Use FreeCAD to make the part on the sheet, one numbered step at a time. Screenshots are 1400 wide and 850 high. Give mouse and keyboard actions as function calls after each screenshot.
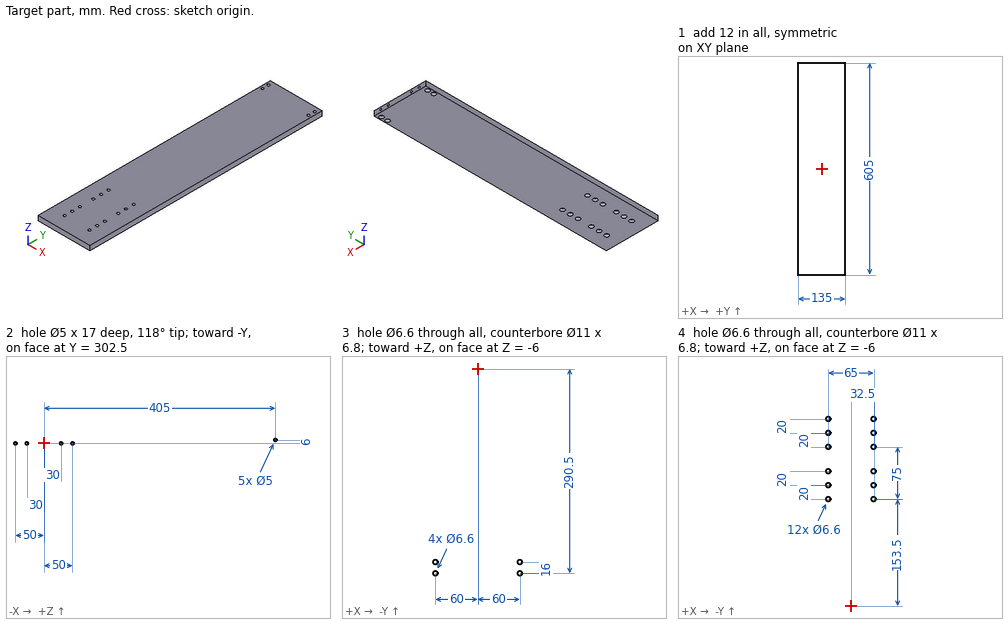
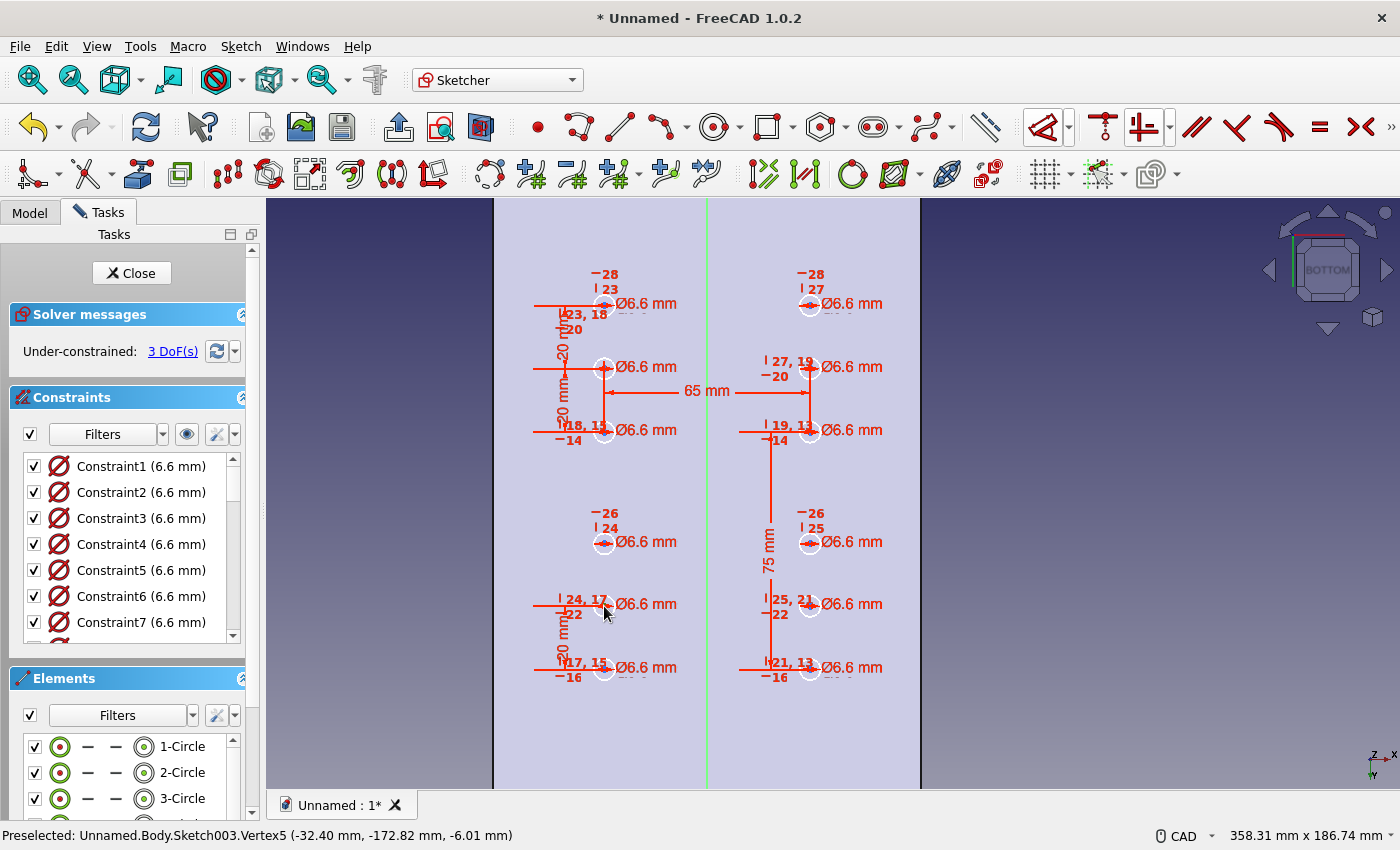
click(604, 544)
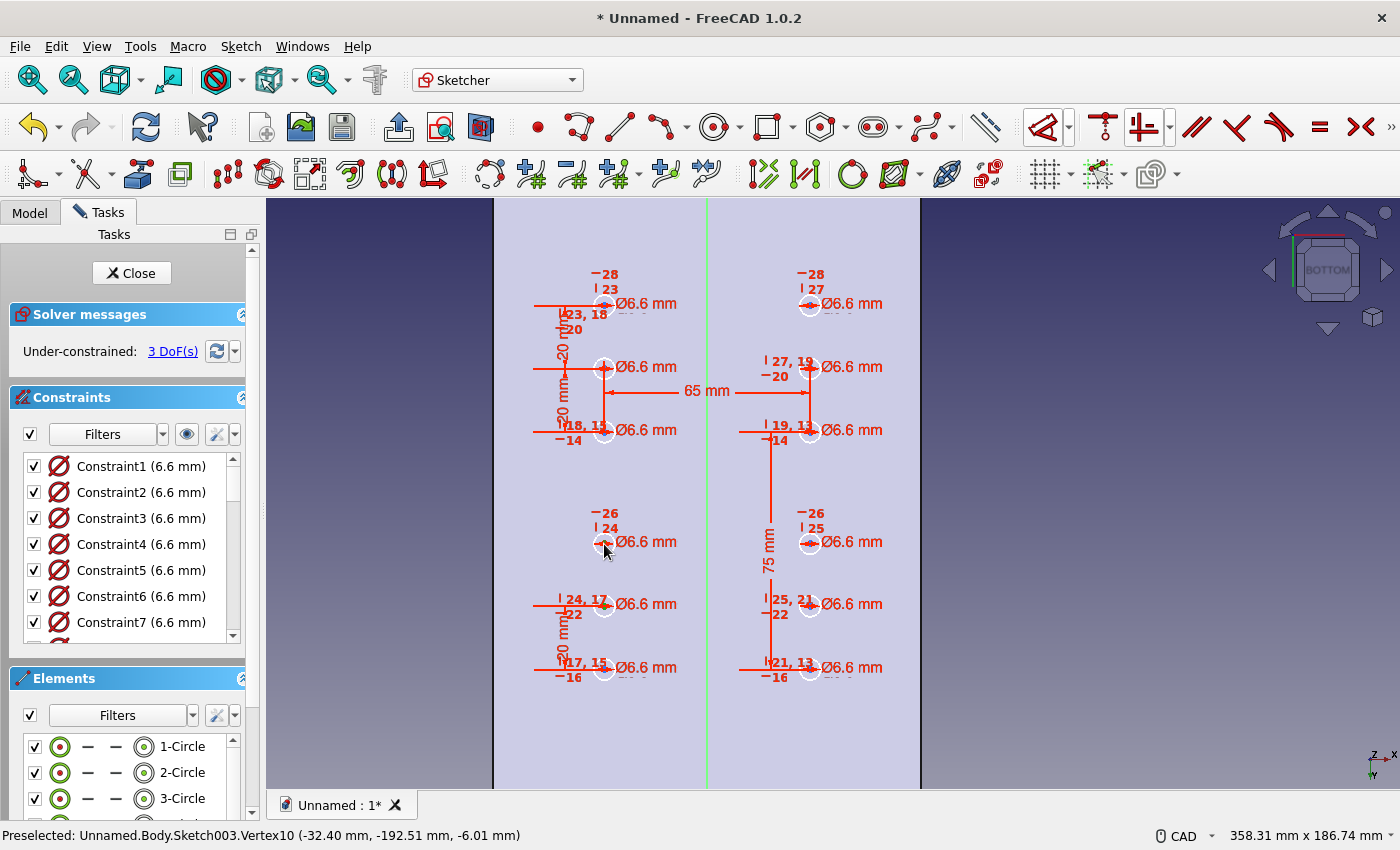
click(1068, 128)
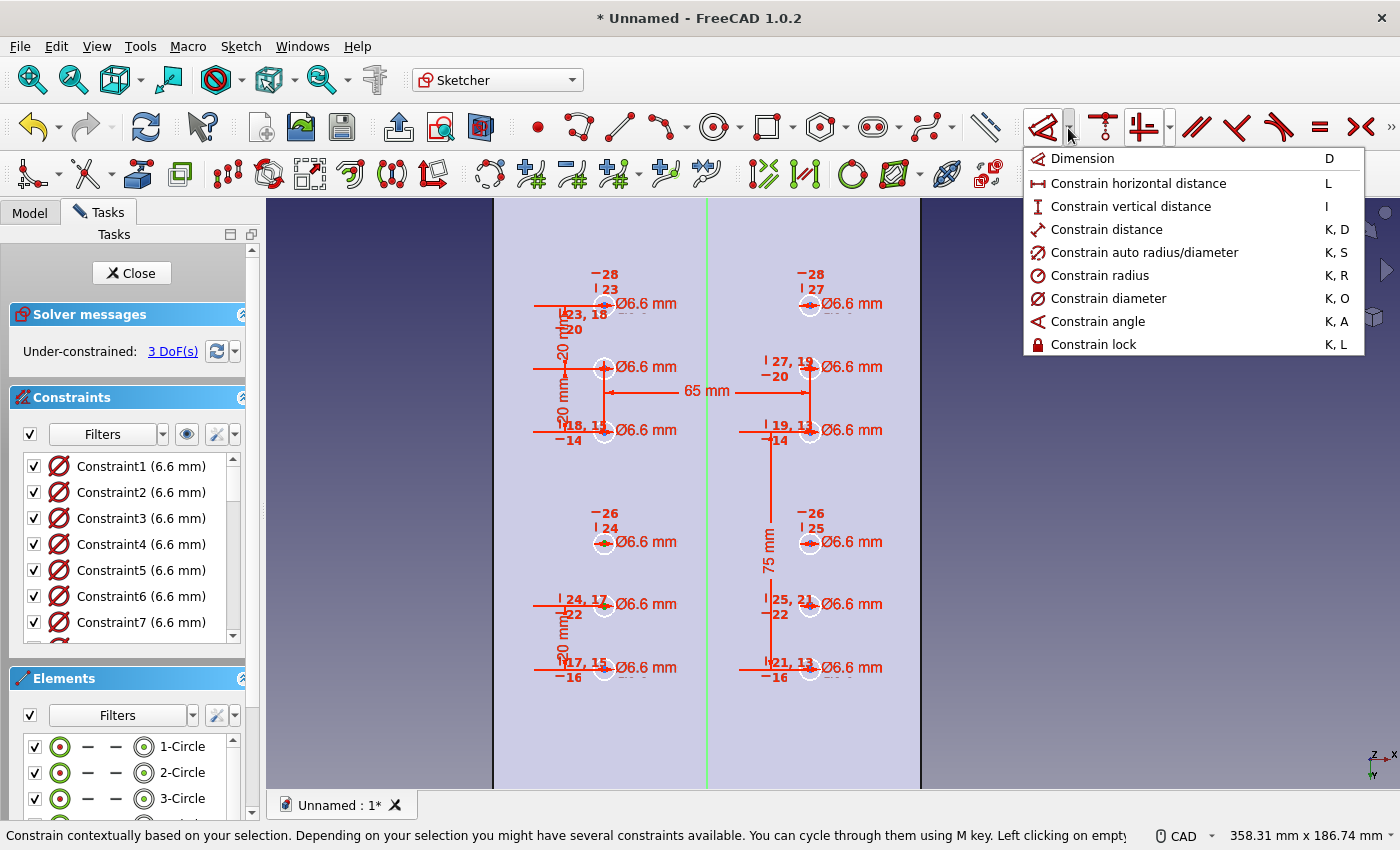
click(1194, 206)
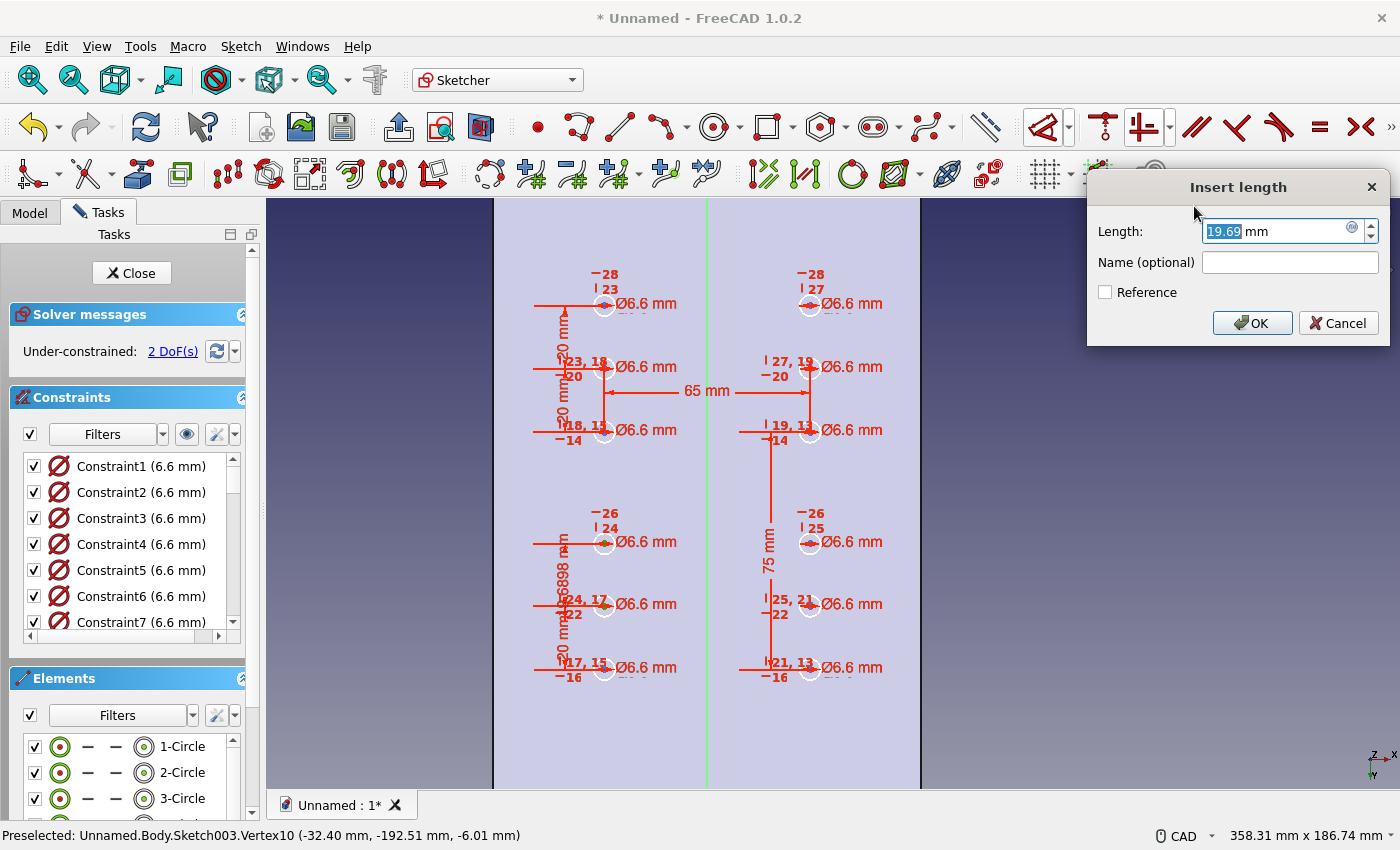
text(20)
key(Return)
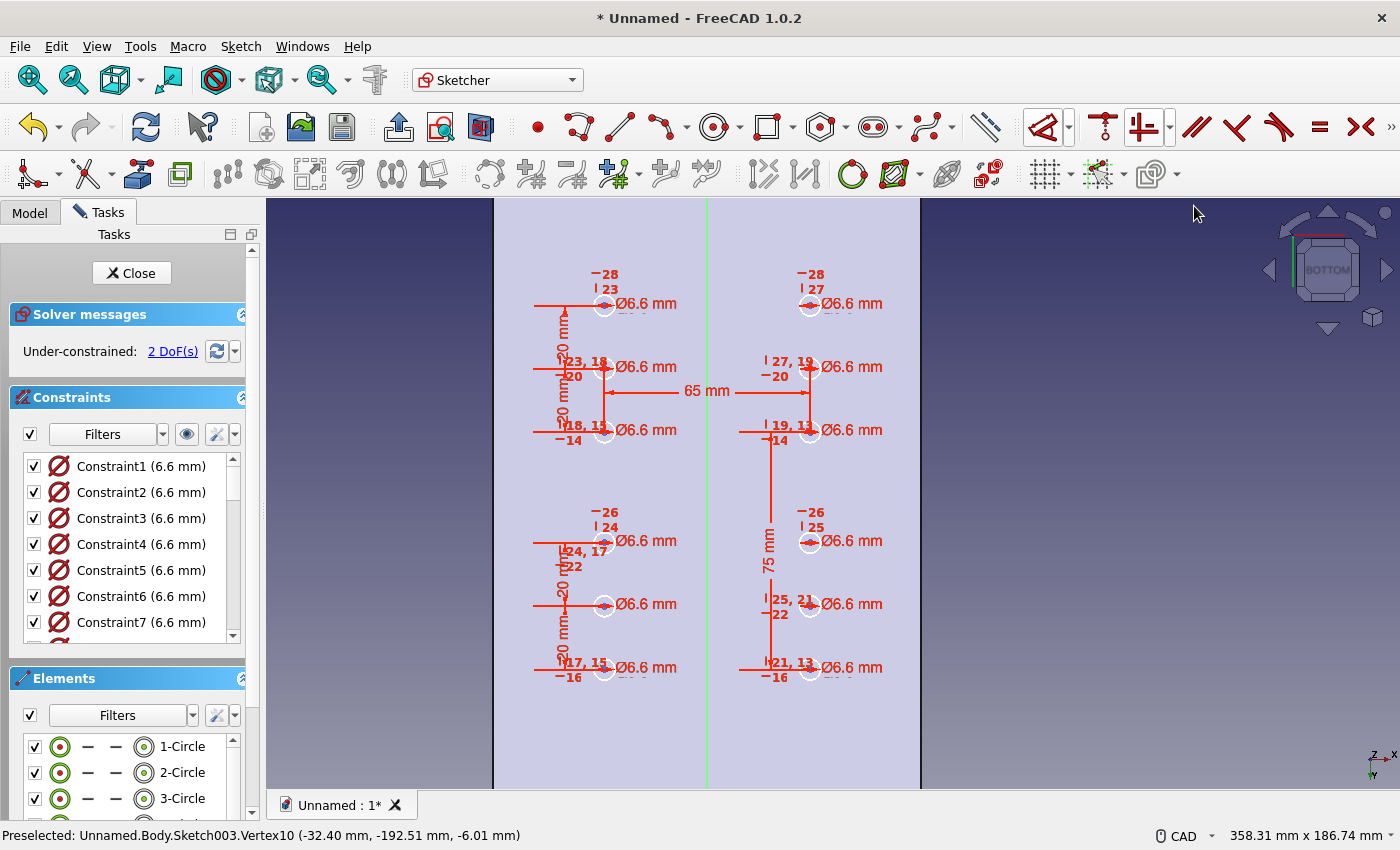
click(810, 670)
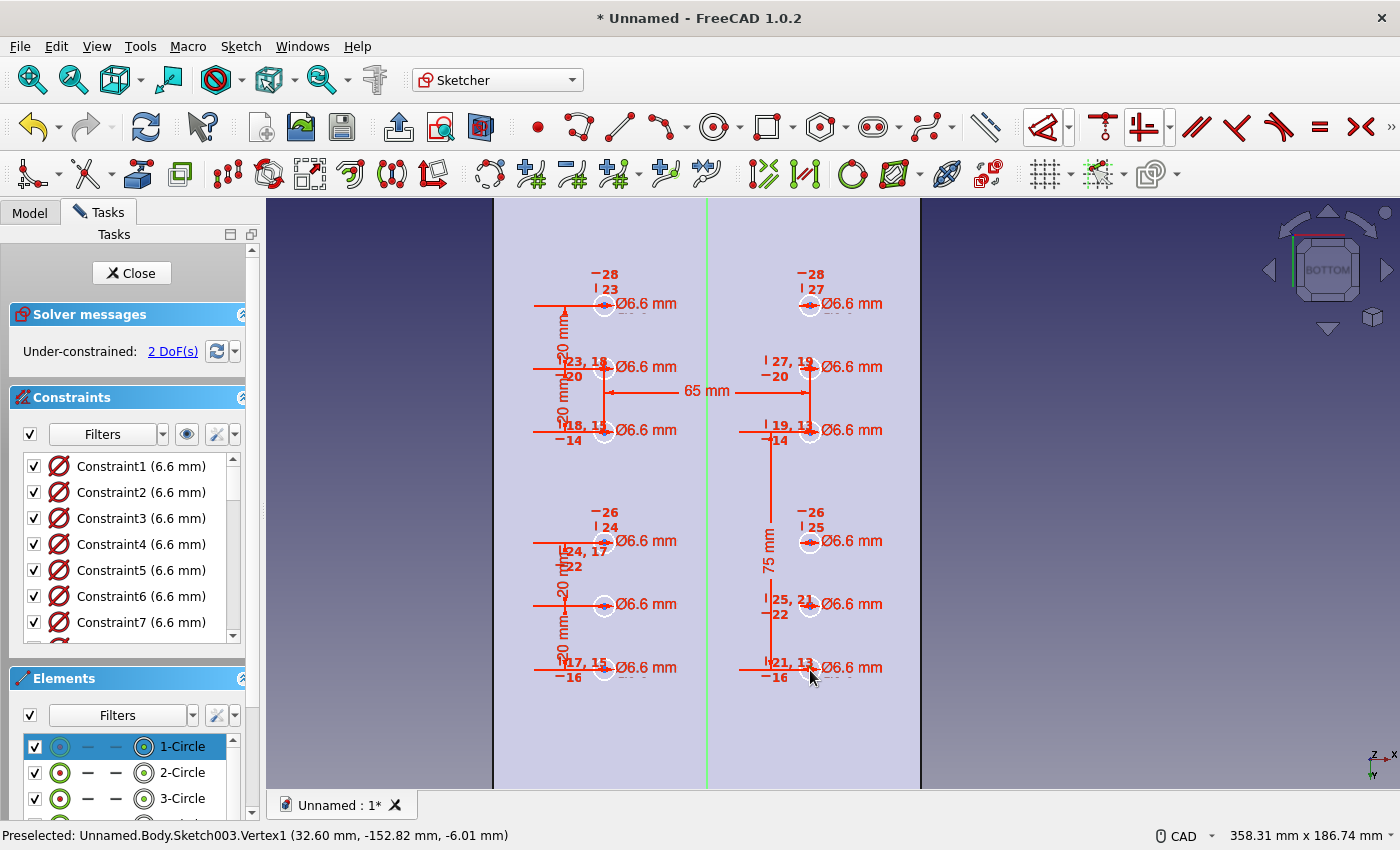
key(l)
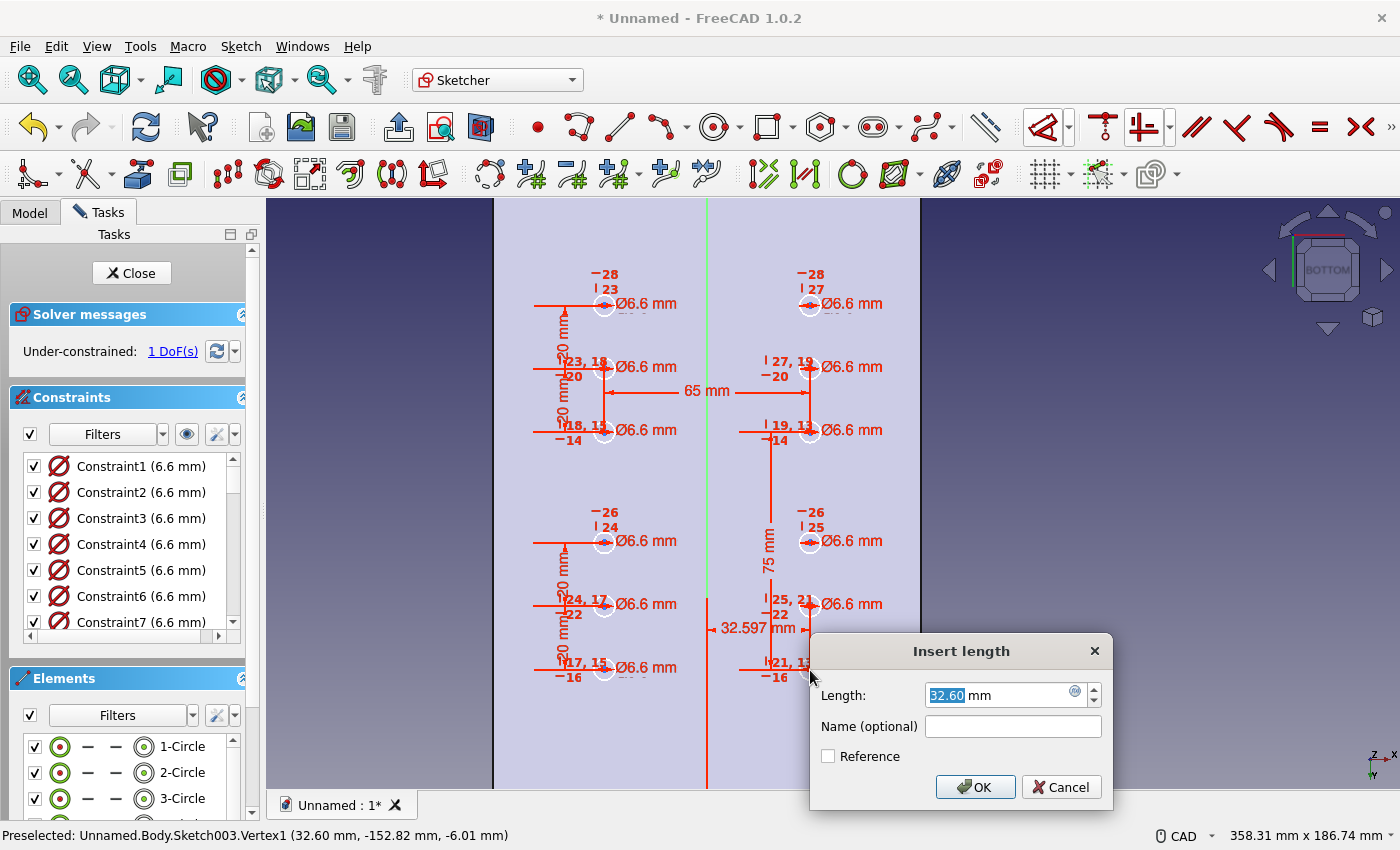
text(32.5)
key(Return)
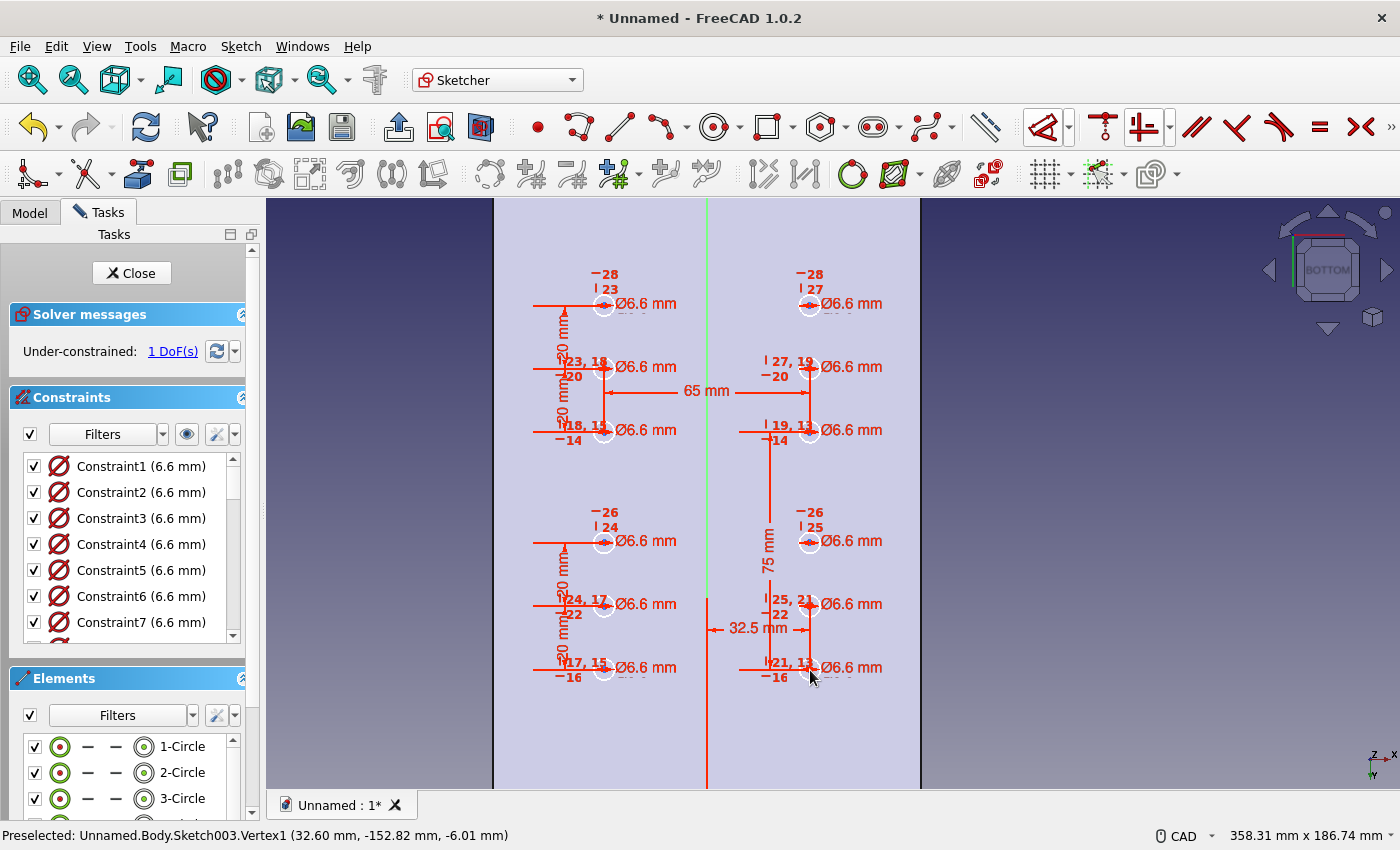
click(810, 670)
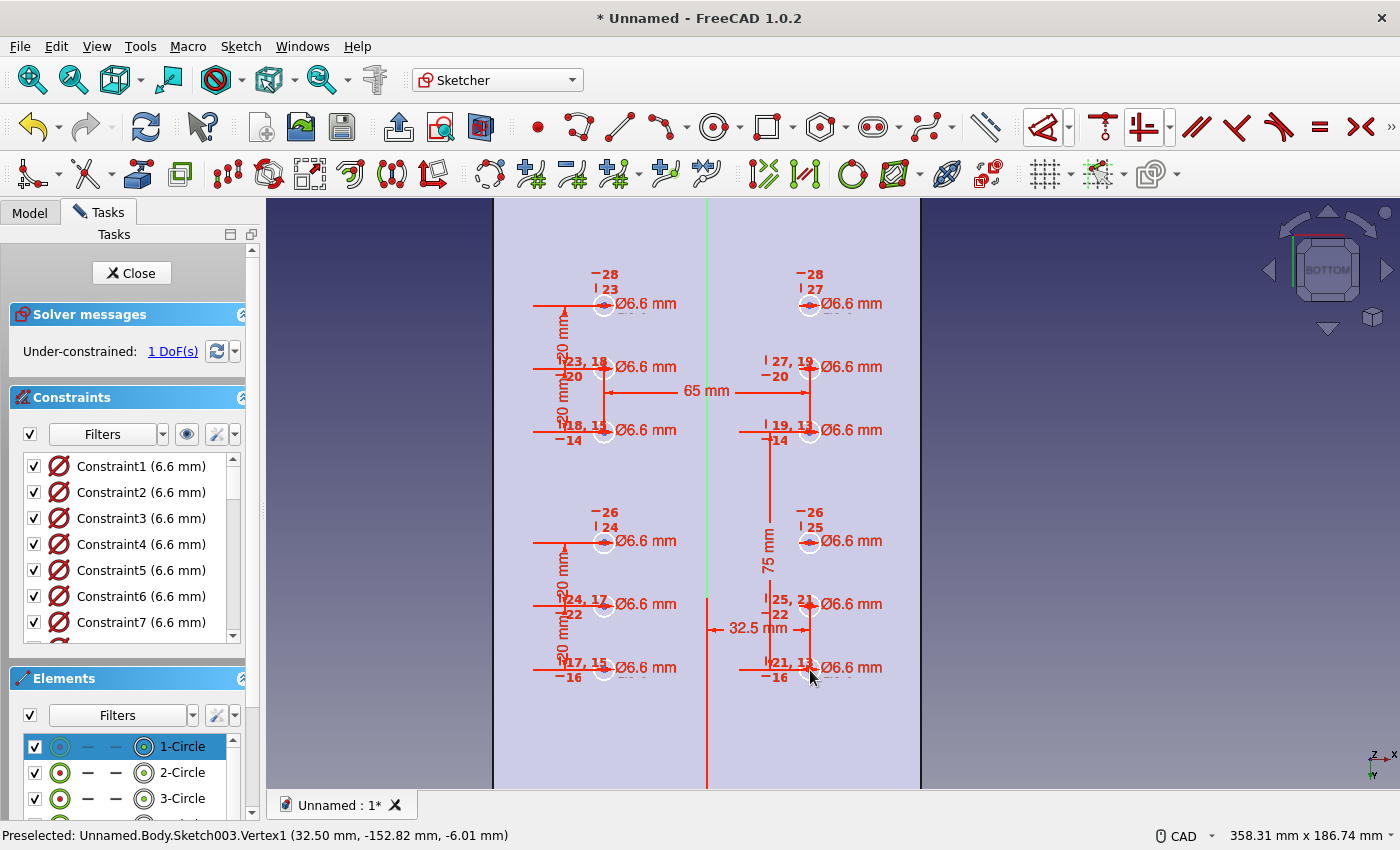
key(i)